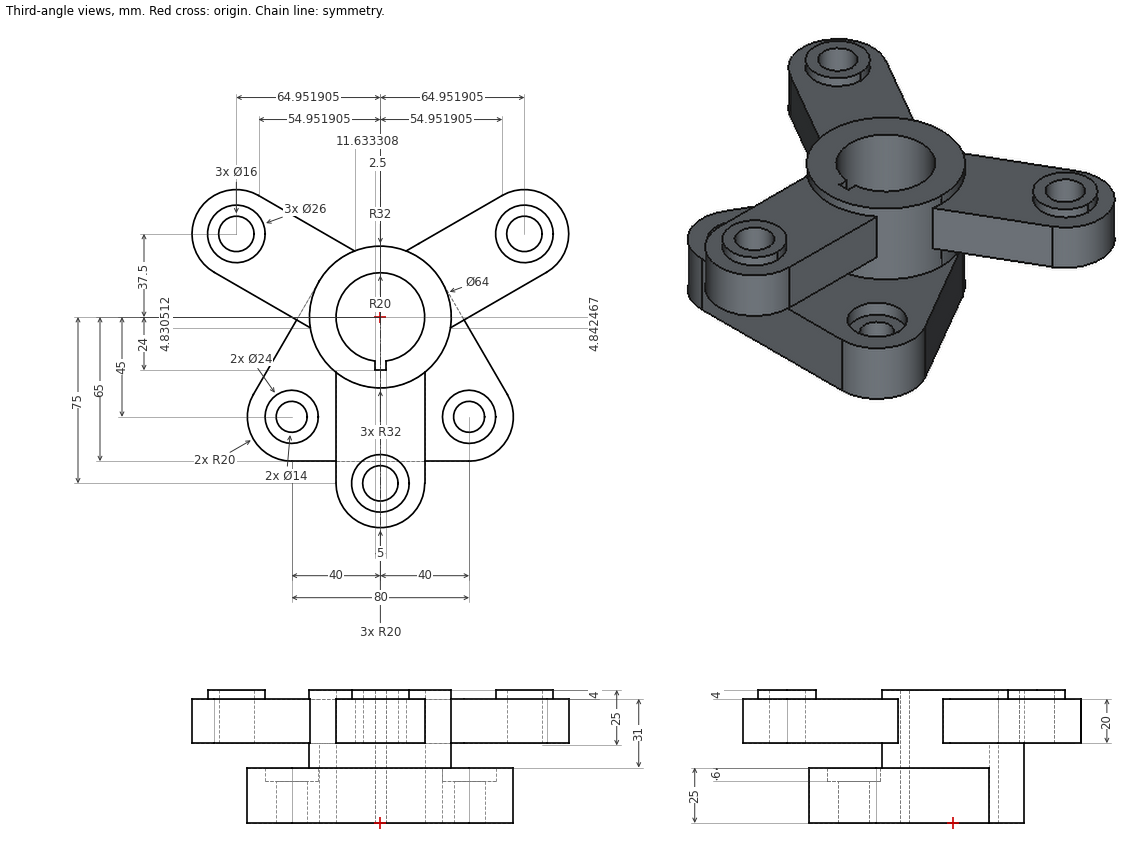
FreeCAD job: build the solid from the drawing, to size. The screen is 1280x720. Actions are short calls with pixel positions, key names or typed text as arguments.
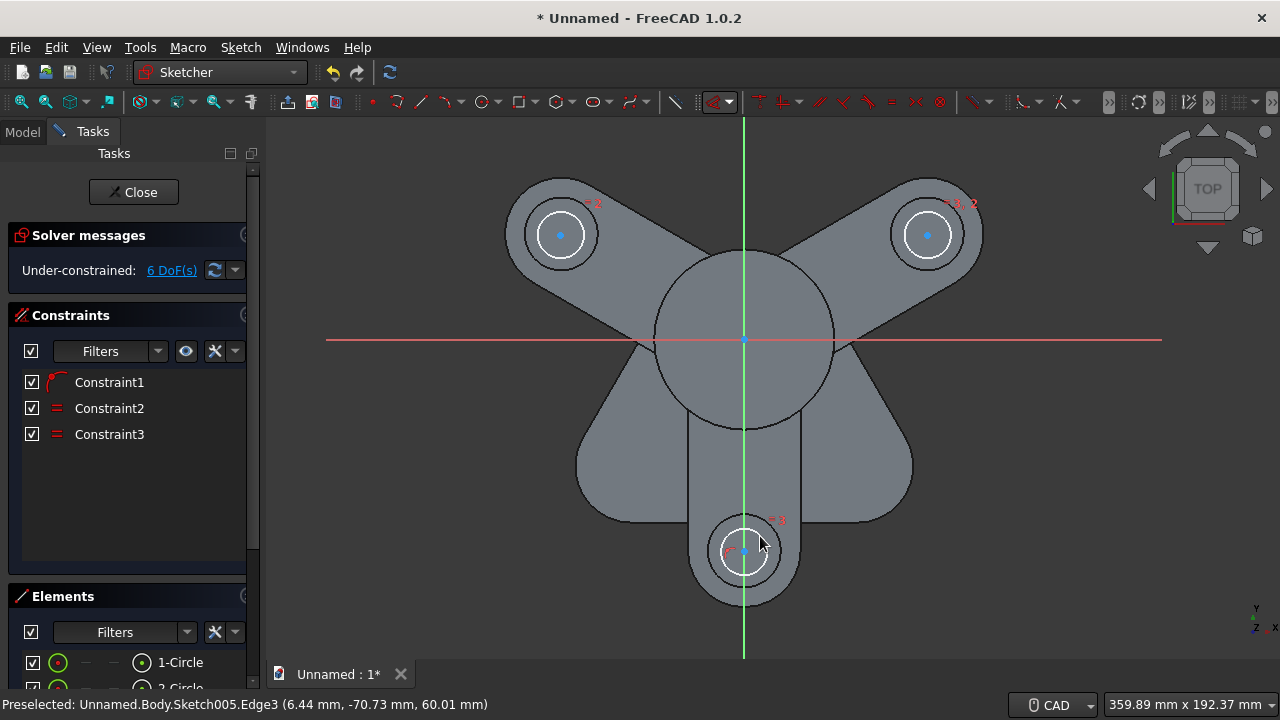
click(561, 235)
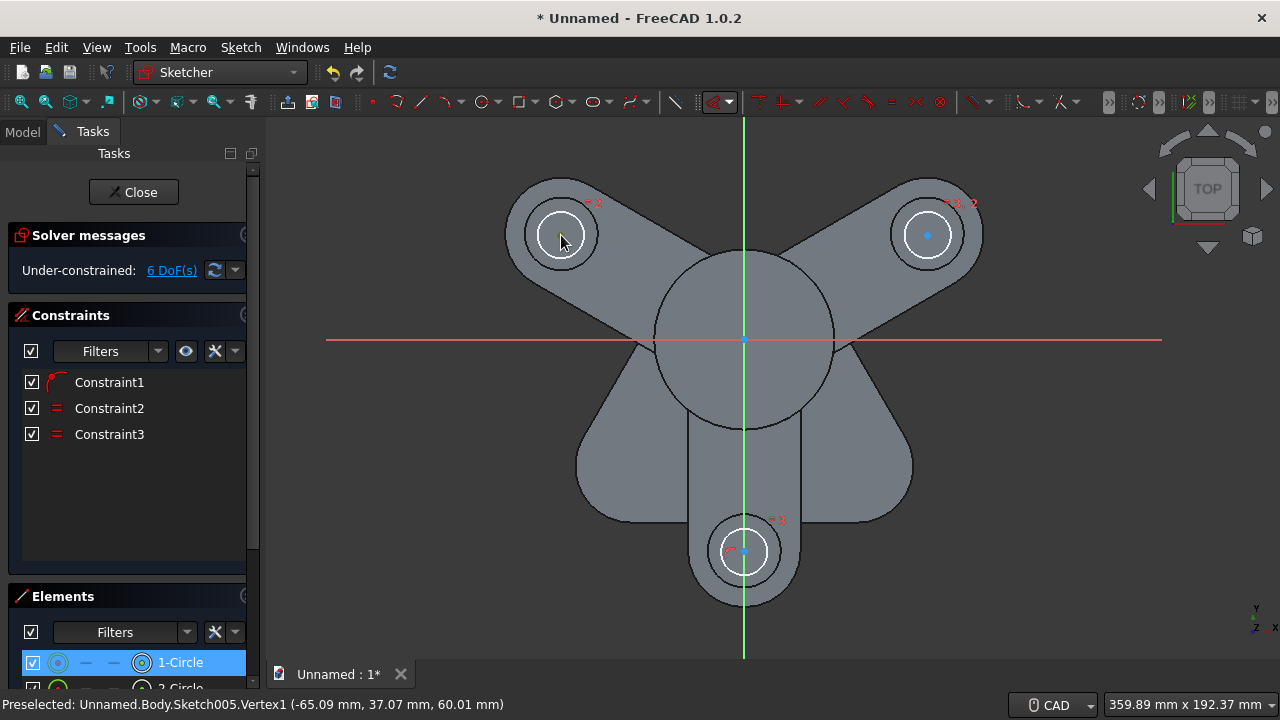
click(928, 235)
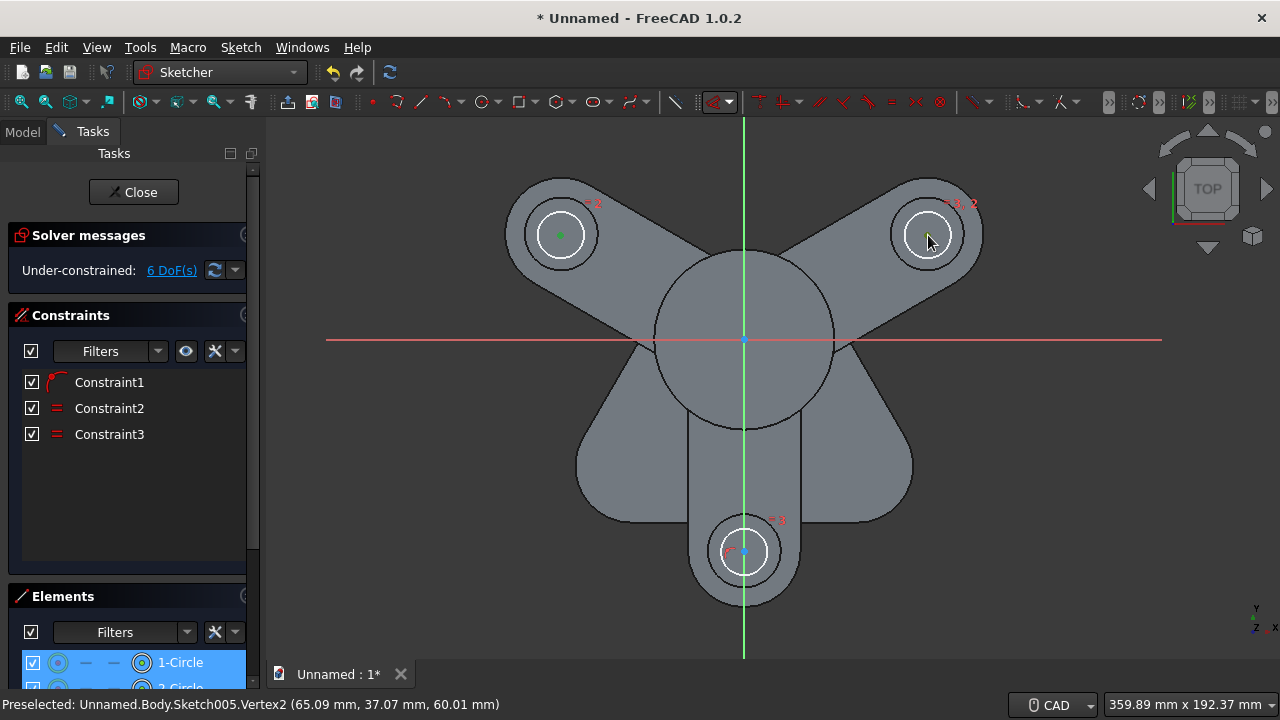
key(h)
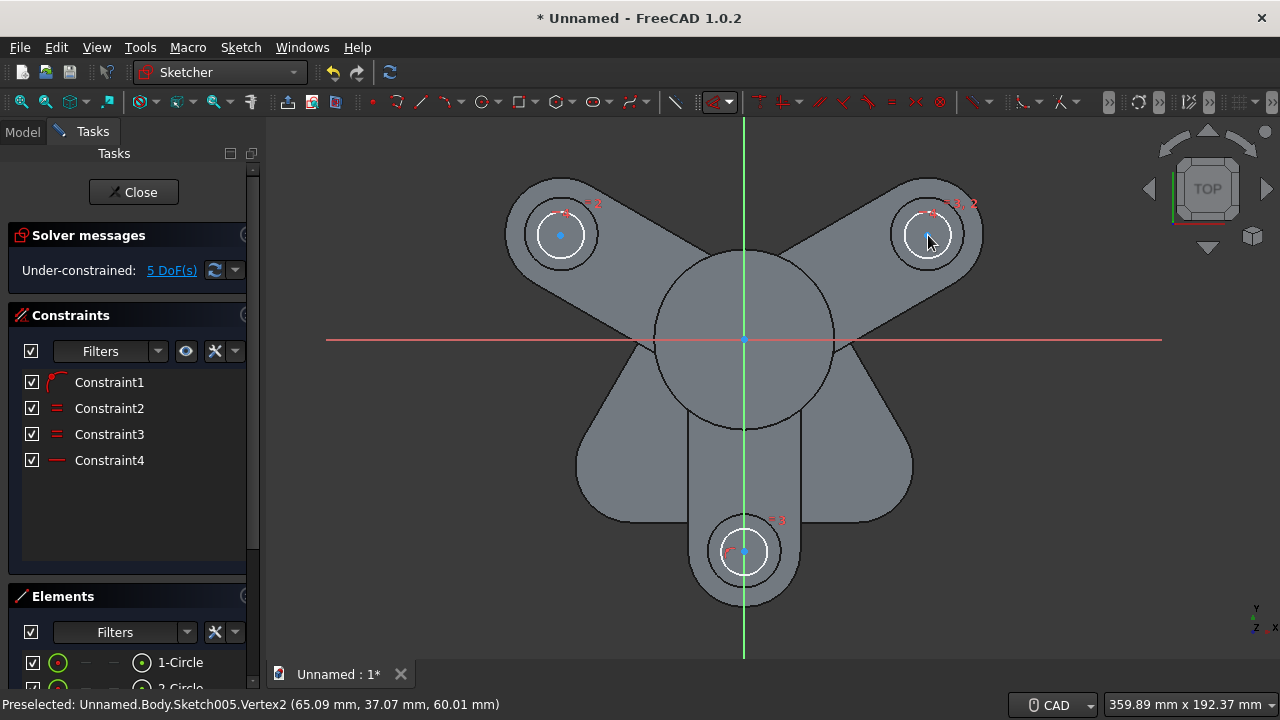
click(577, 219)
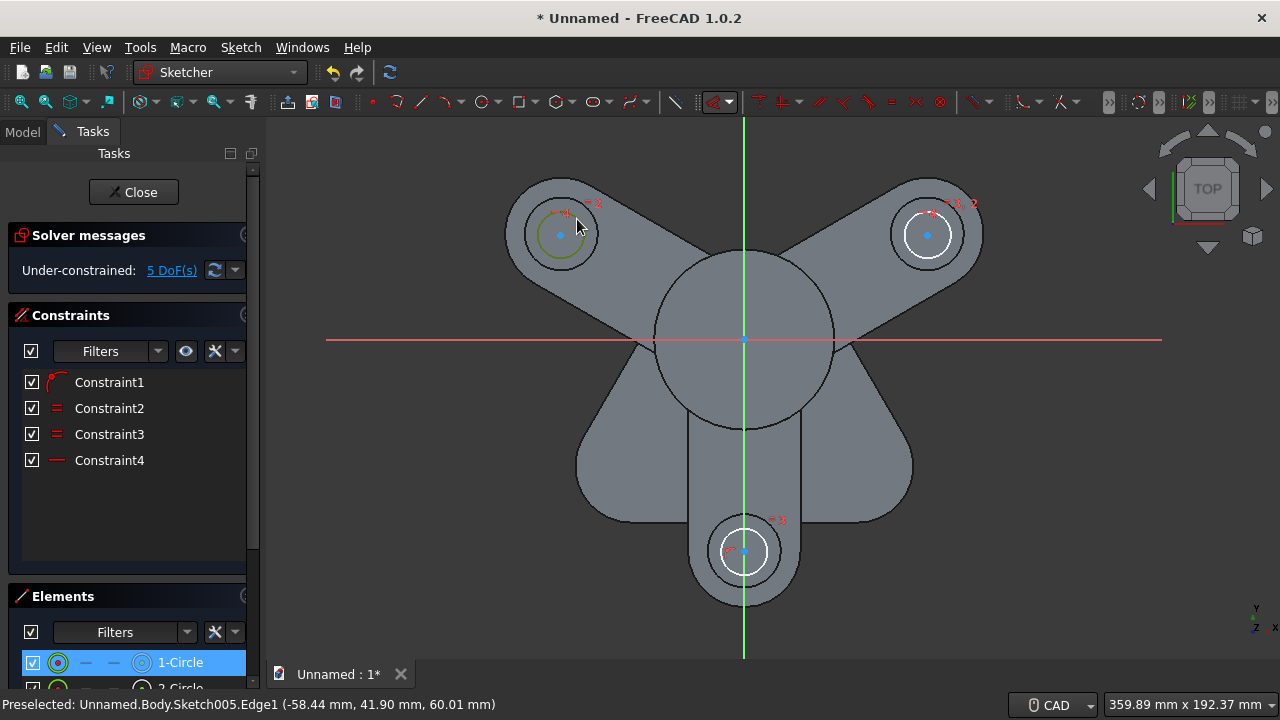
key(k)
key(o)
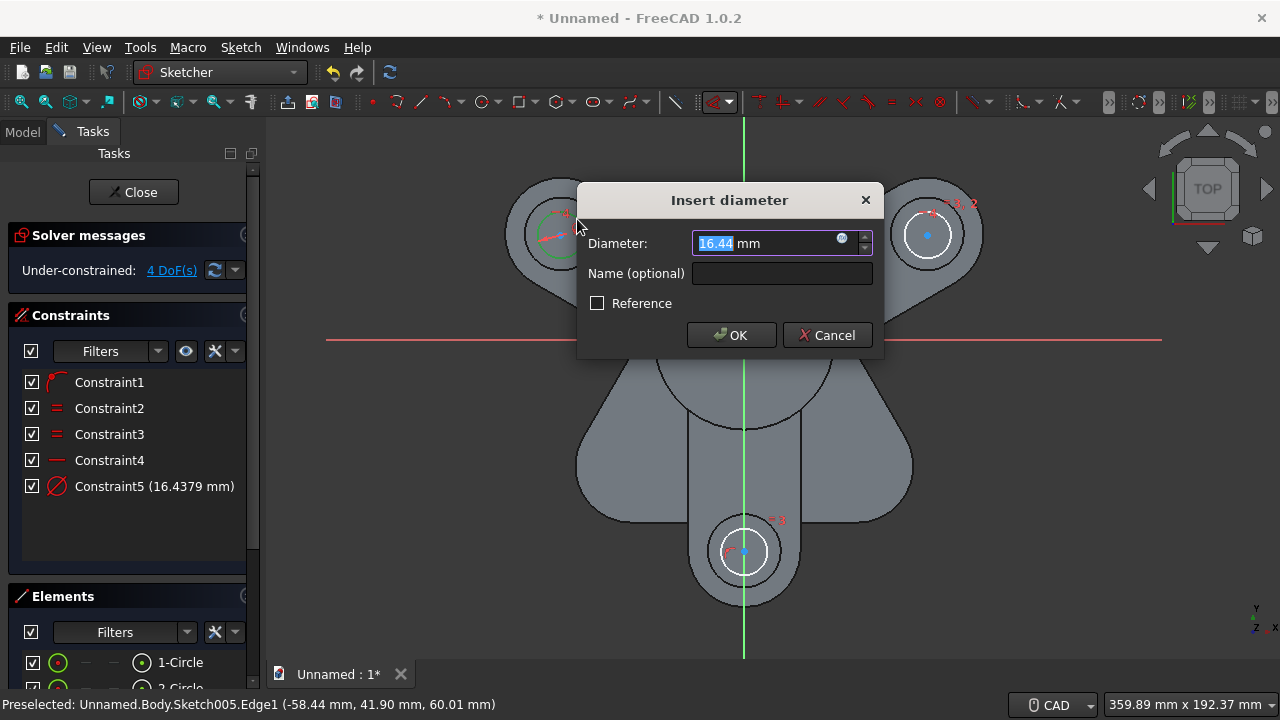
text(16)
key(Return)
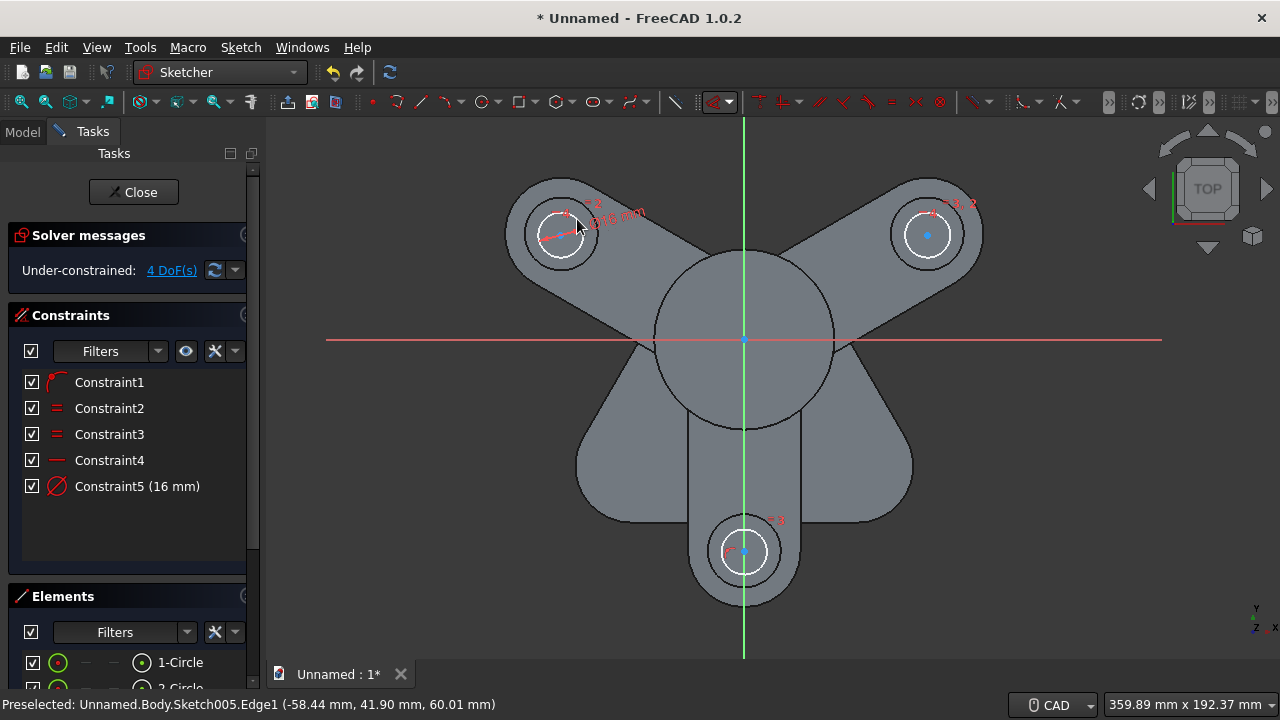
click(744, 552)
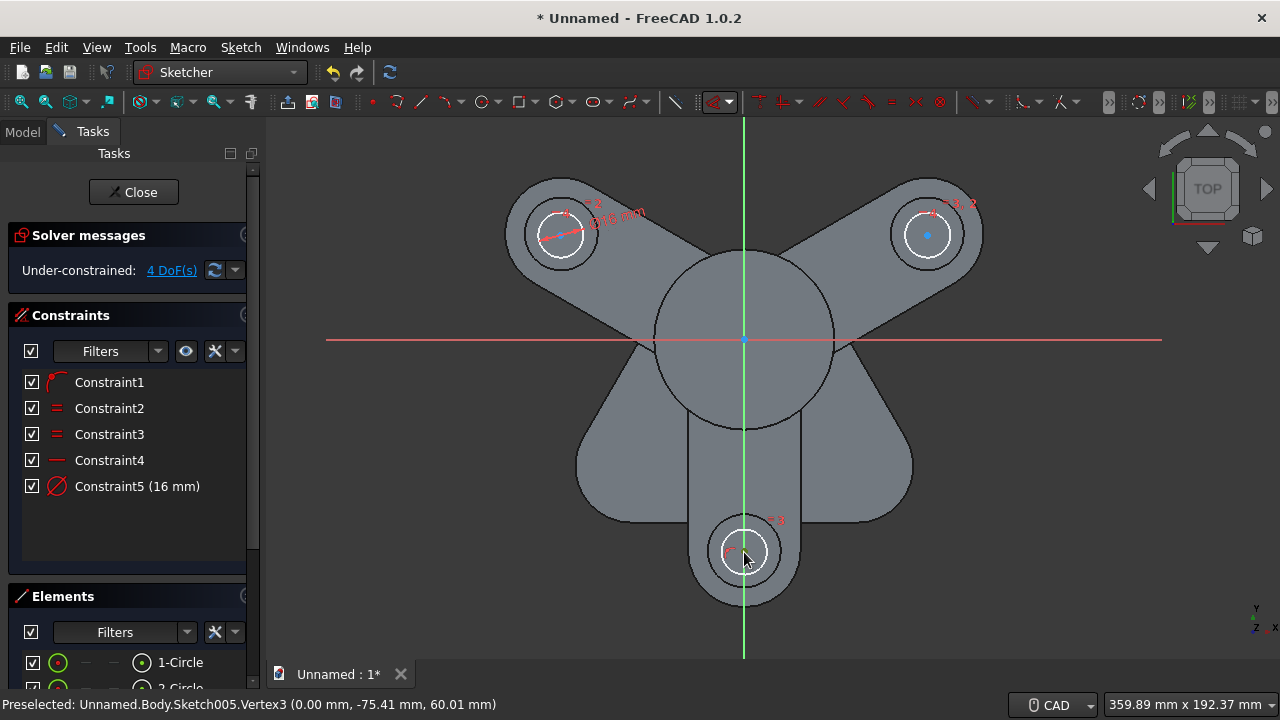
click(732, 102)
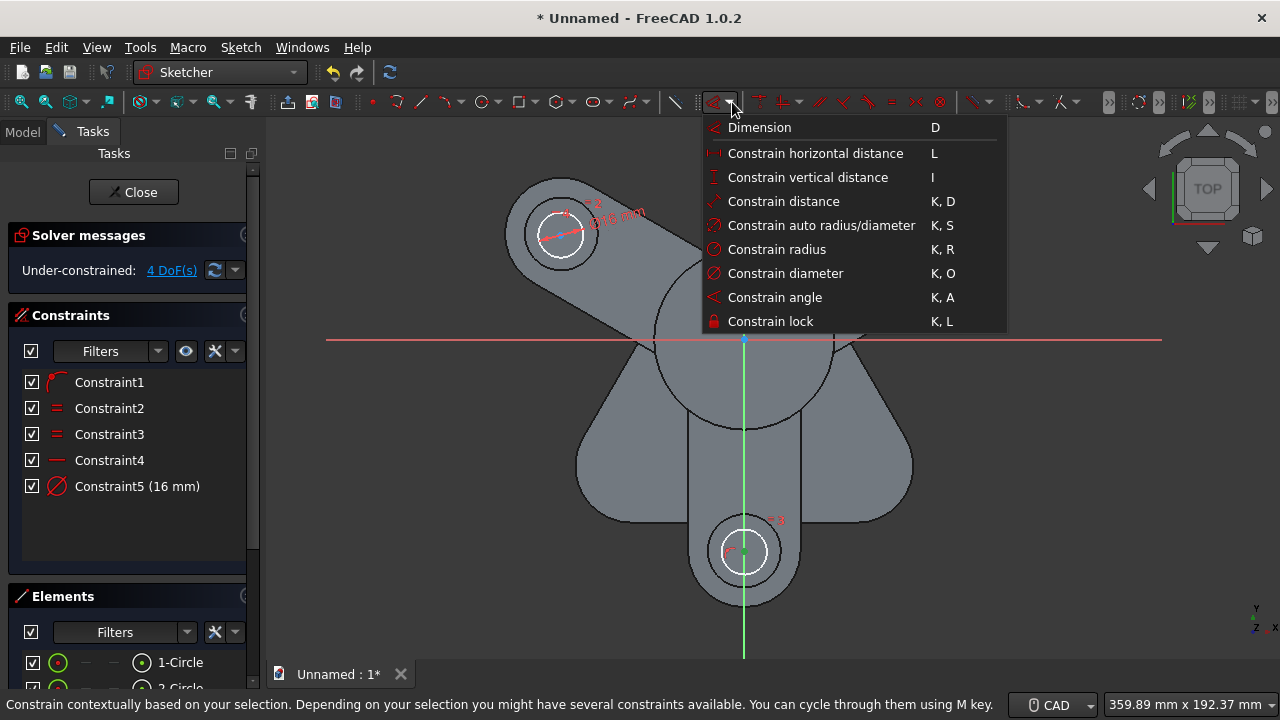
click(855, 177)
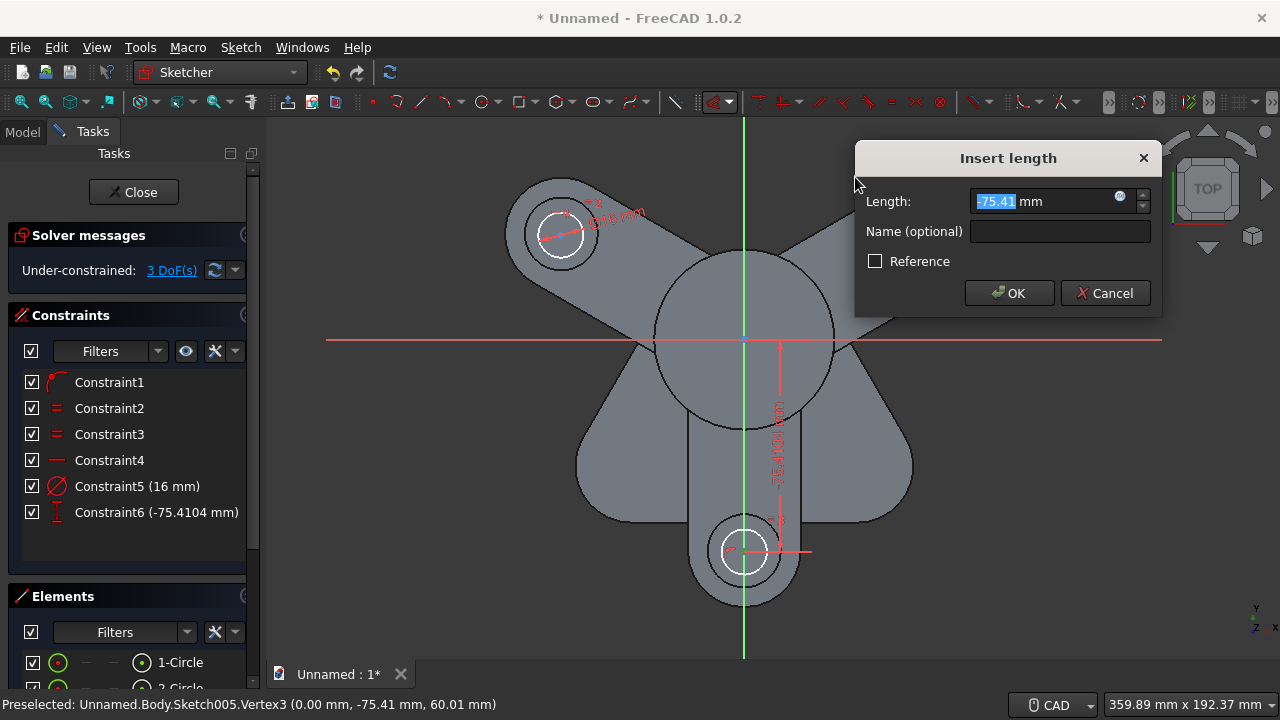
text(-75)
key(Return)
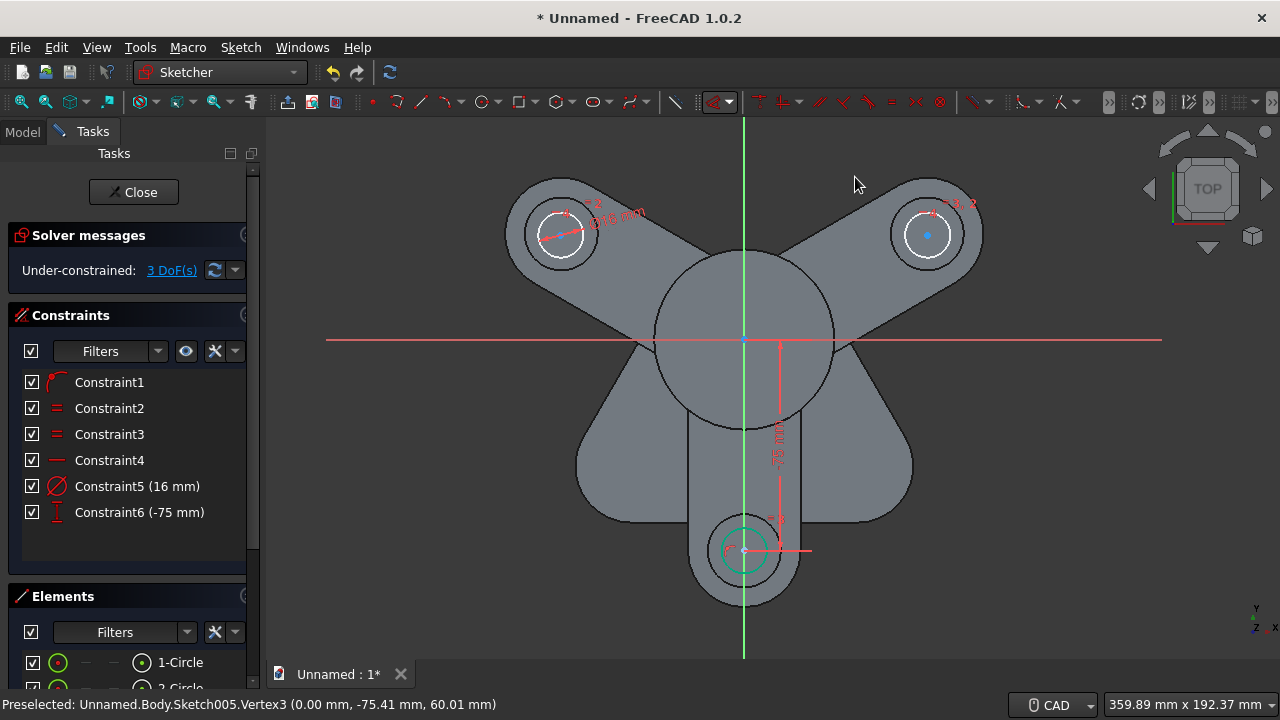
click(561, 235)